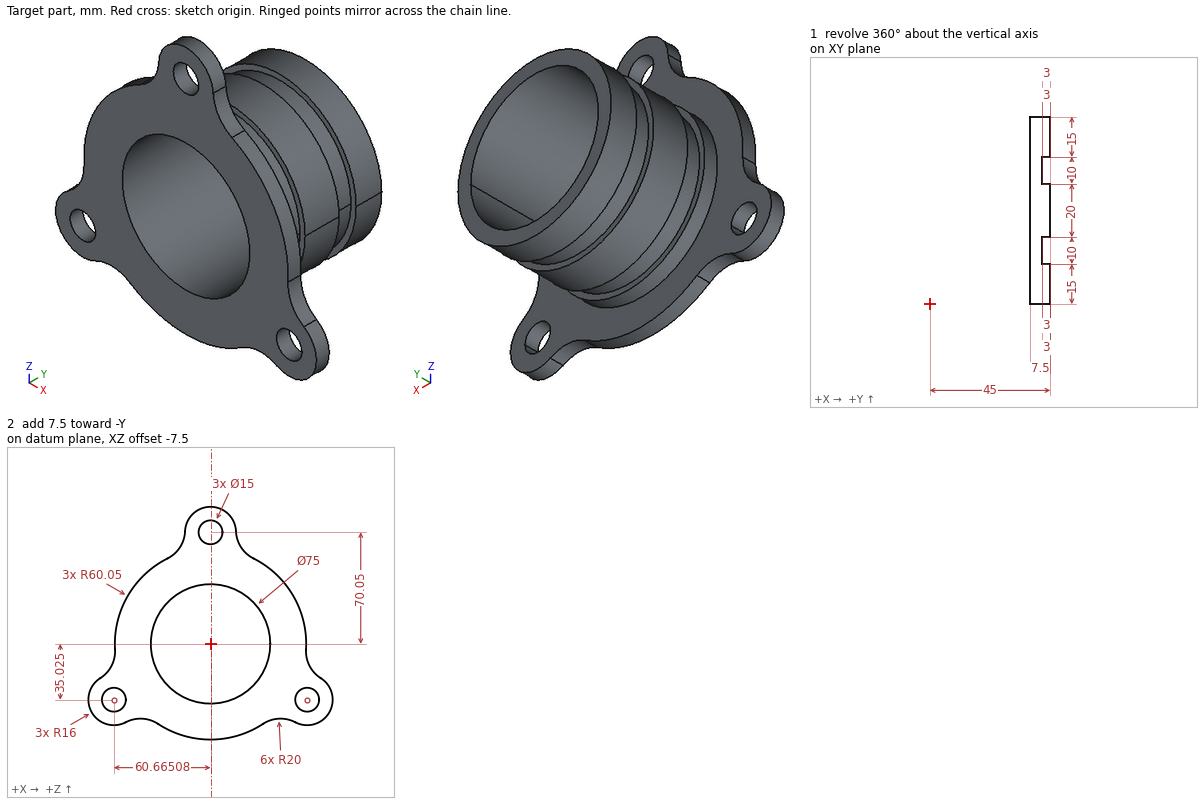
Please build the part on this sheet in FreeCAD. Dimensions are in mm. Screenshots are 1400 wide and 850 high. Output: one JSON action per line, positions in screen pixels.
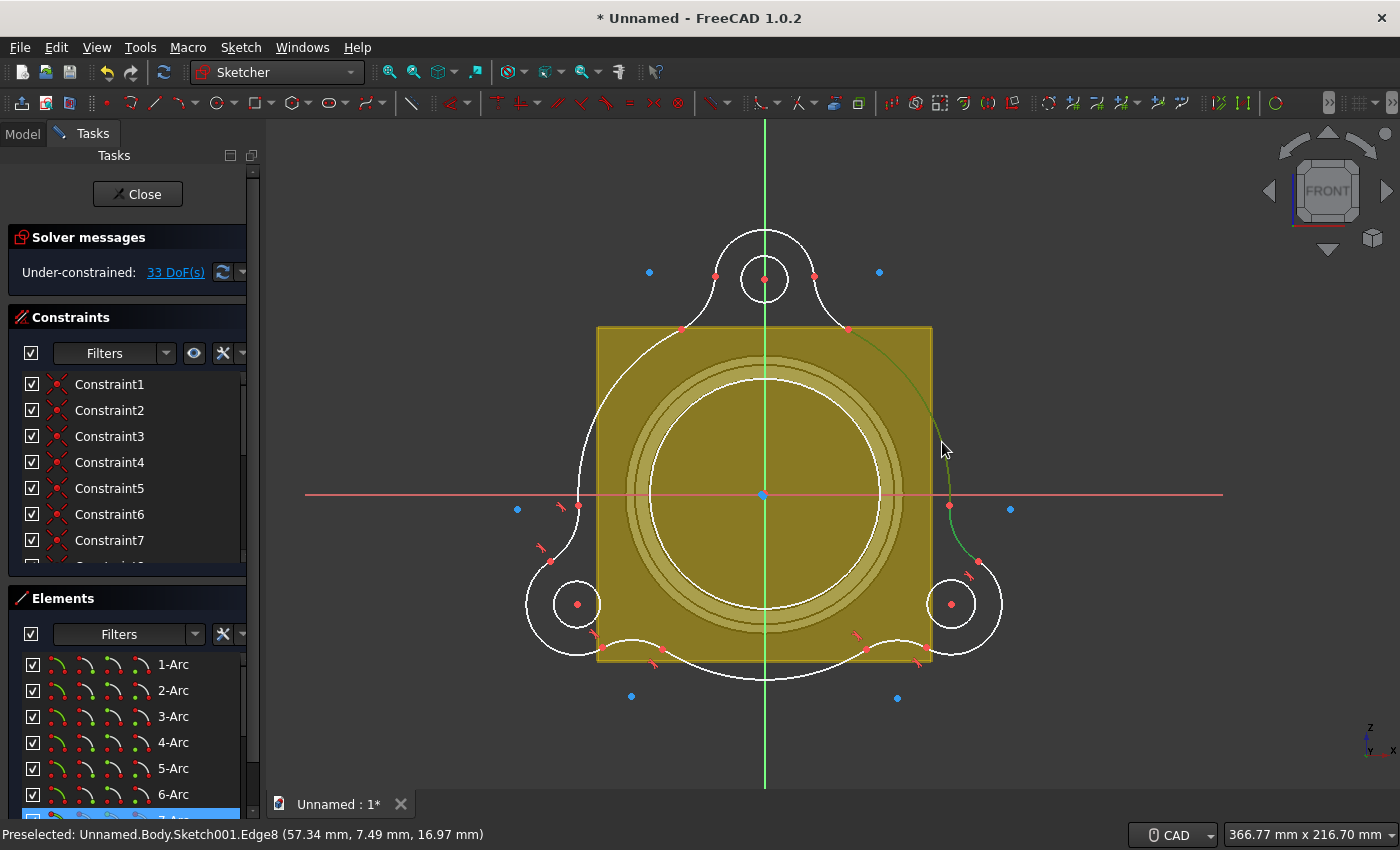
{"action": "left_click", "coordinate": [606, 104]}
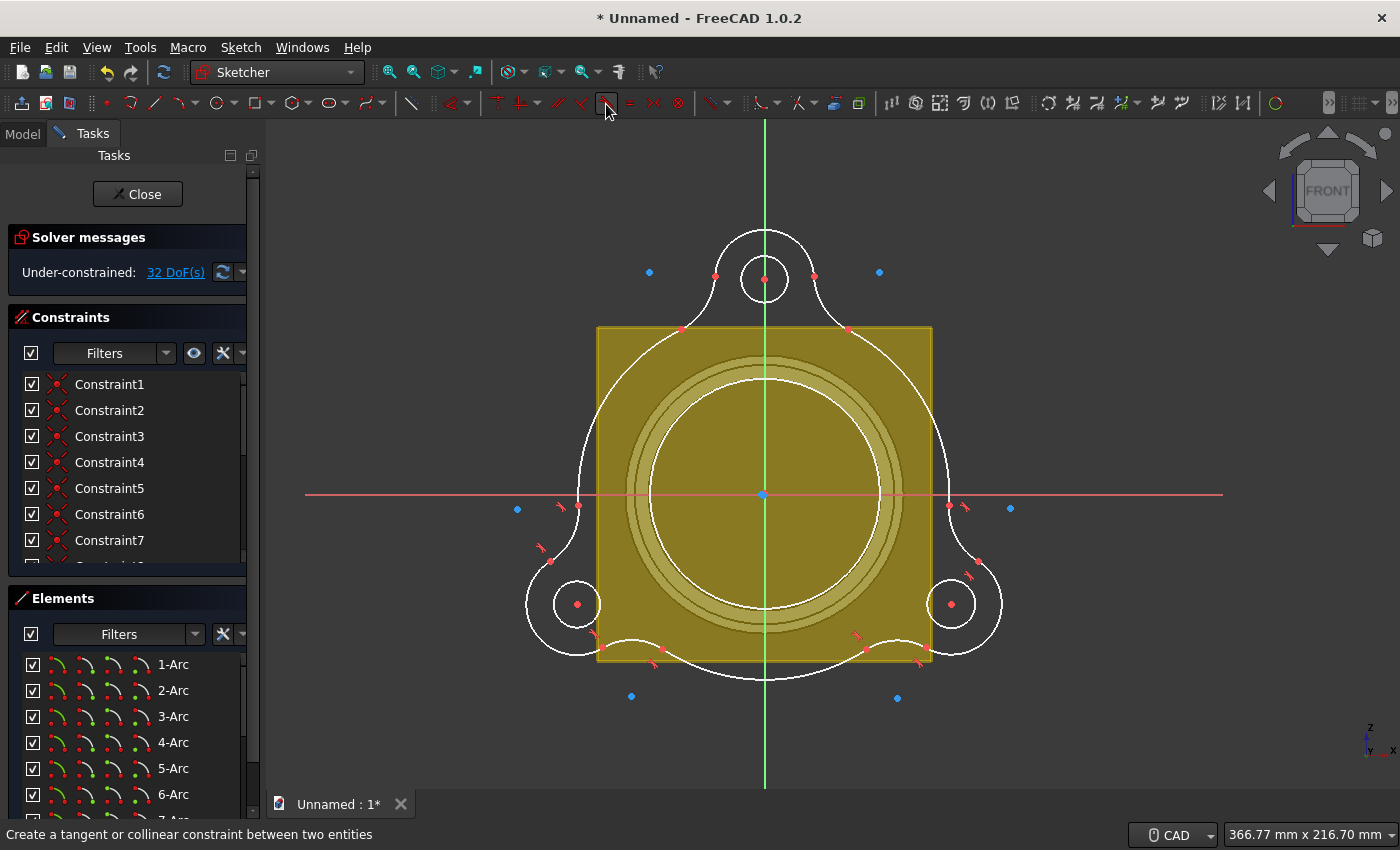
{"action": "left_click", "coordinate": [942, 442]}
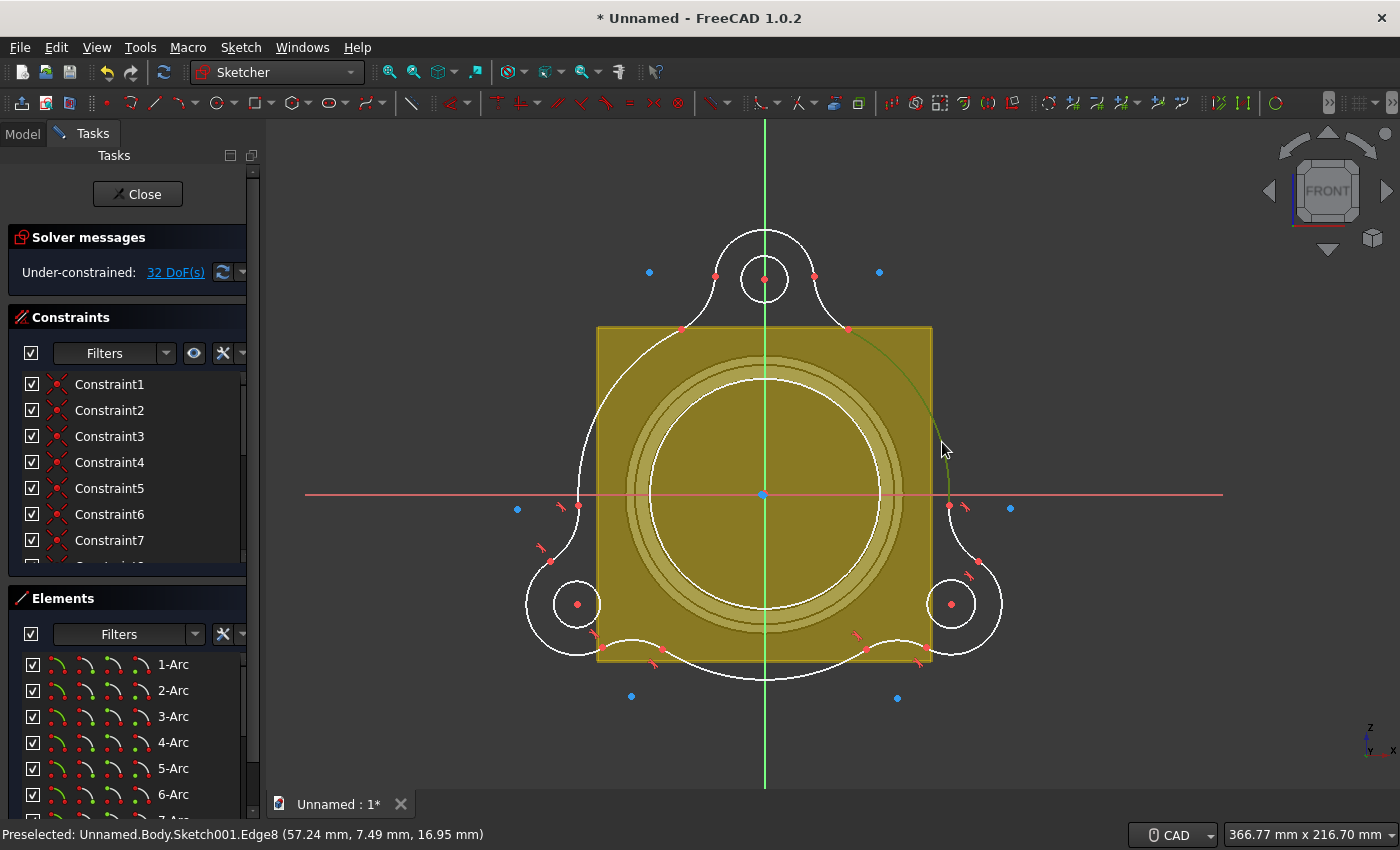
{"action": "left_click", "coordinate": [818, 296]}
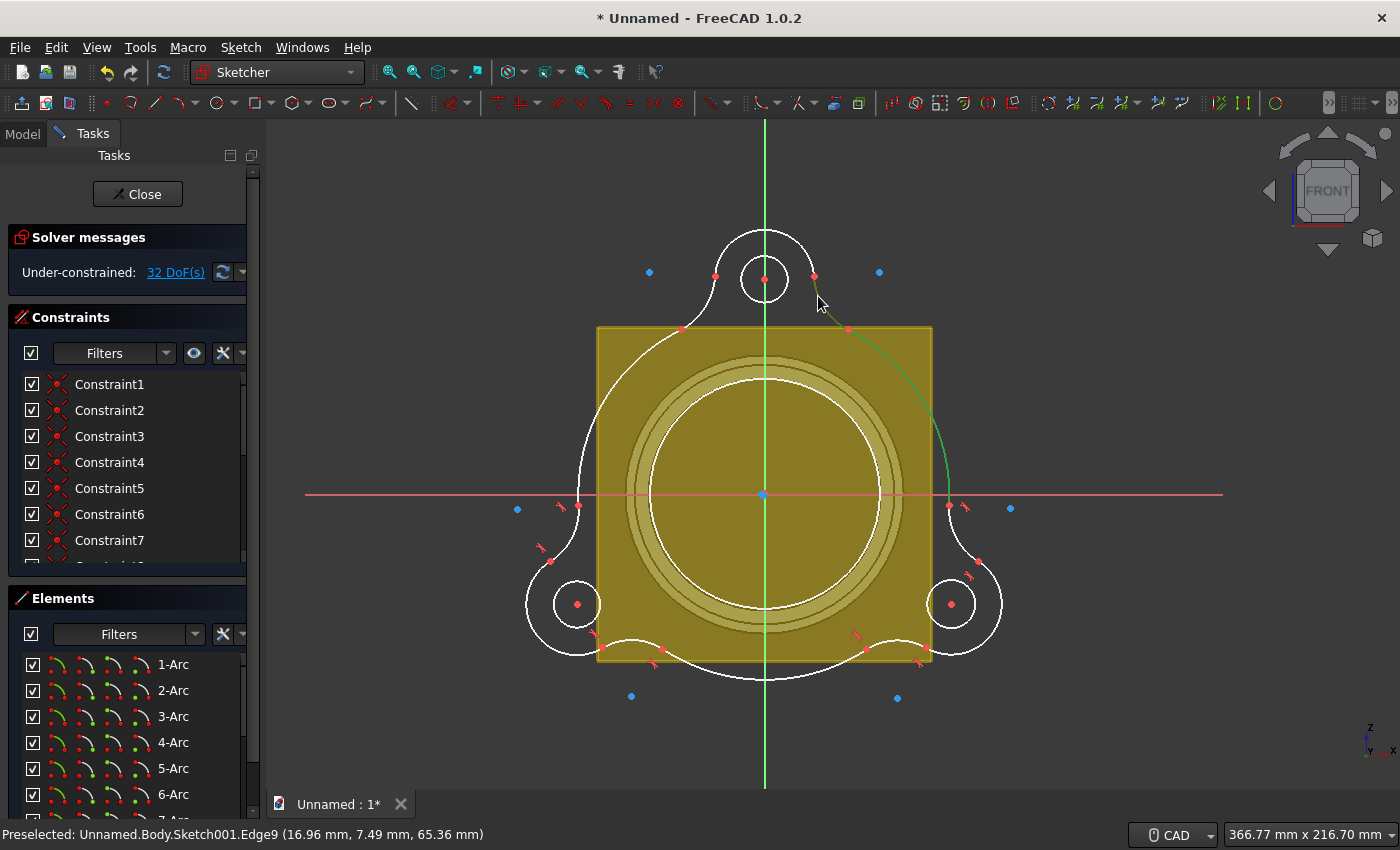
{"action": "left_click", "coordinate": [606, 104]}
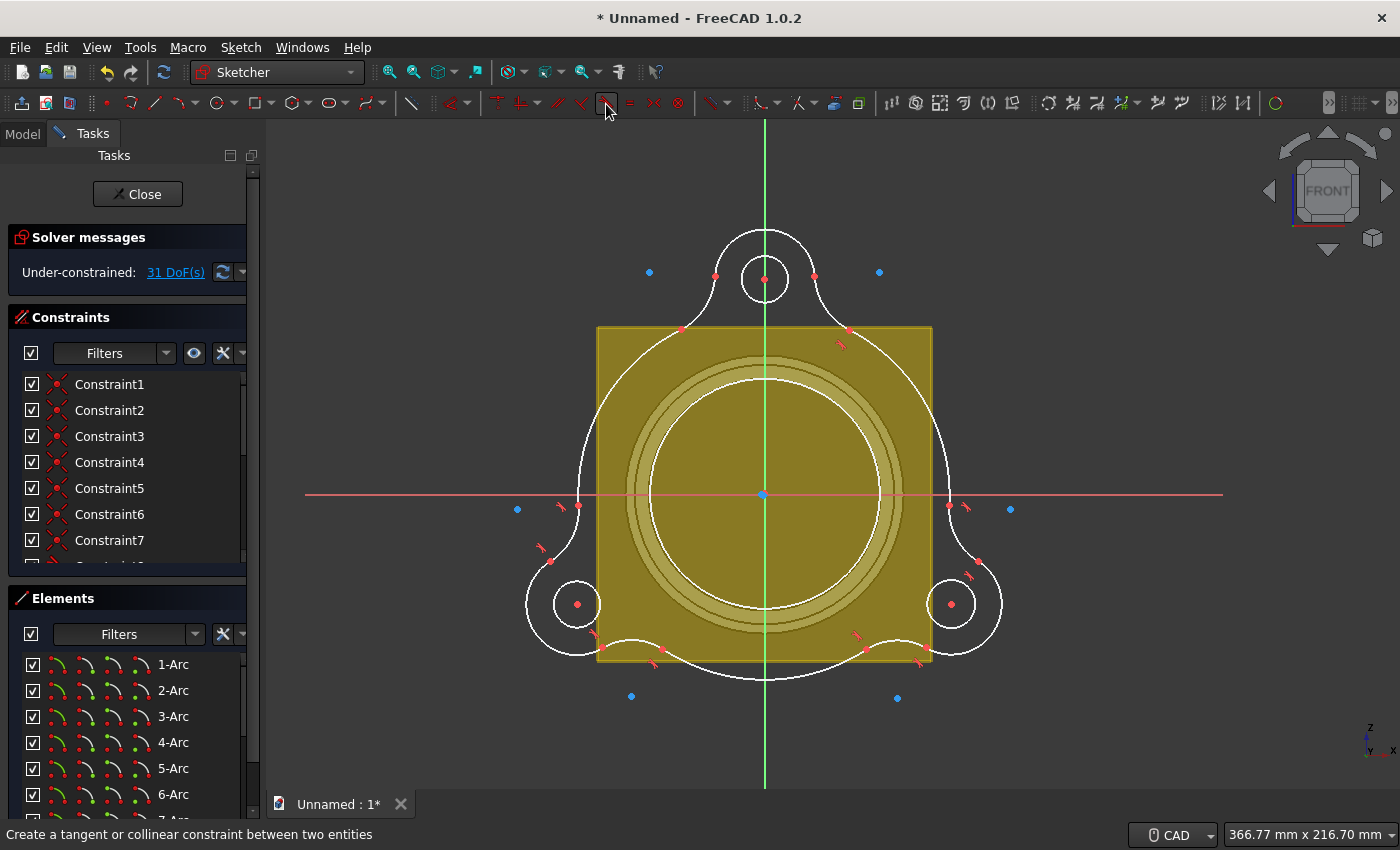
{"action": "left_click", "coordinate": [819, 296]}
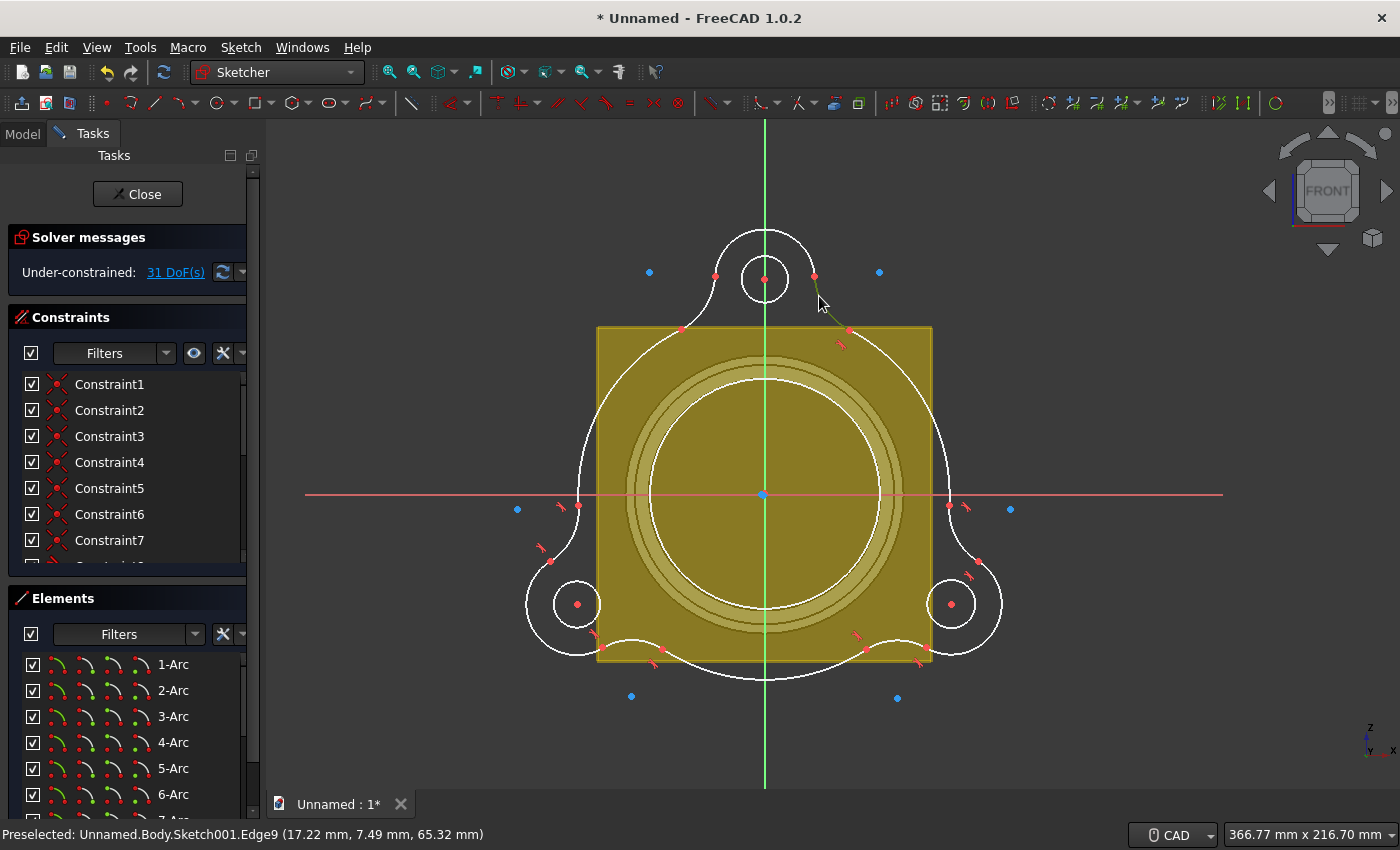
{"action": "left_click", "coordinate": [794, 239]}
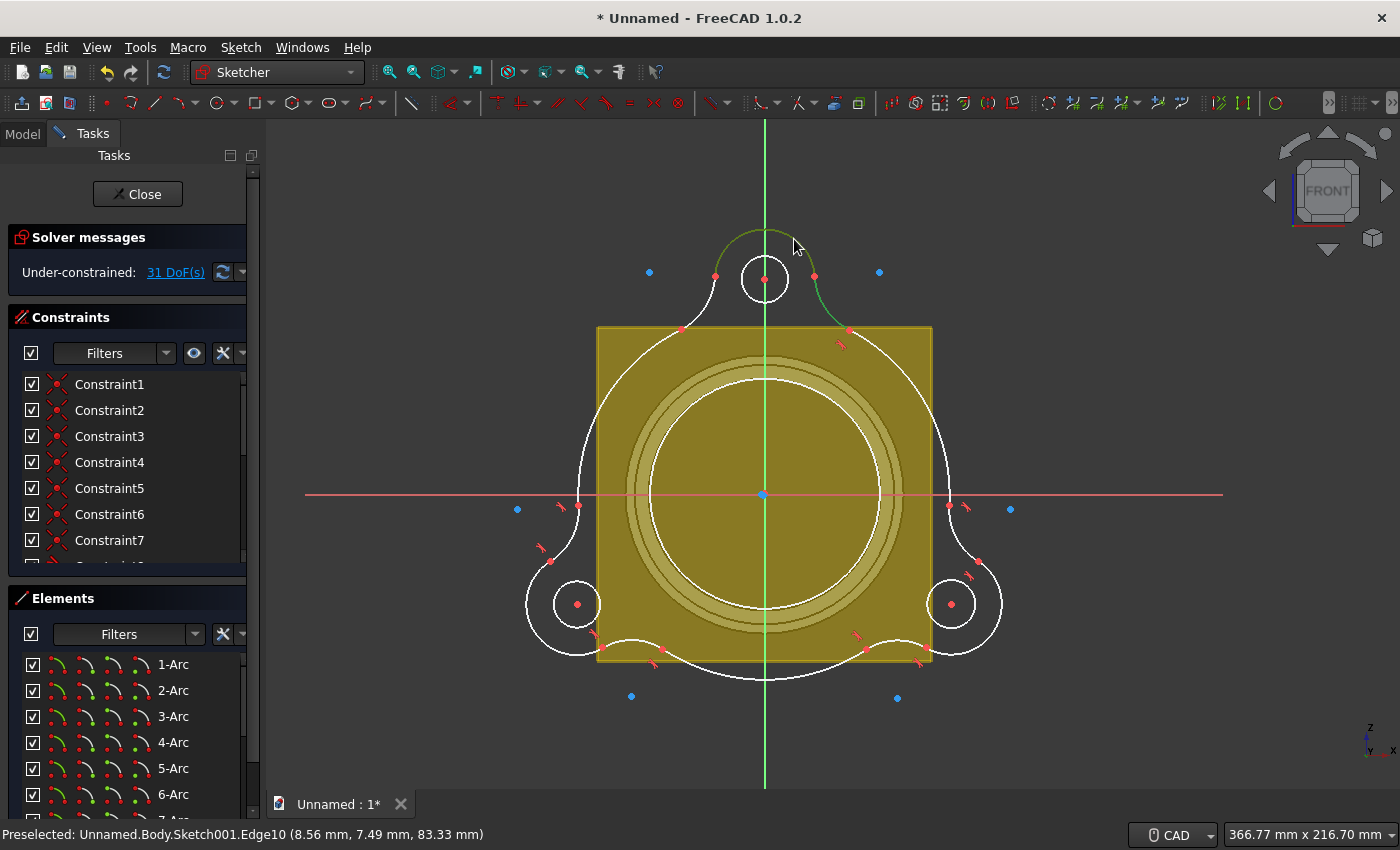
{"action": "key", "text": "t"}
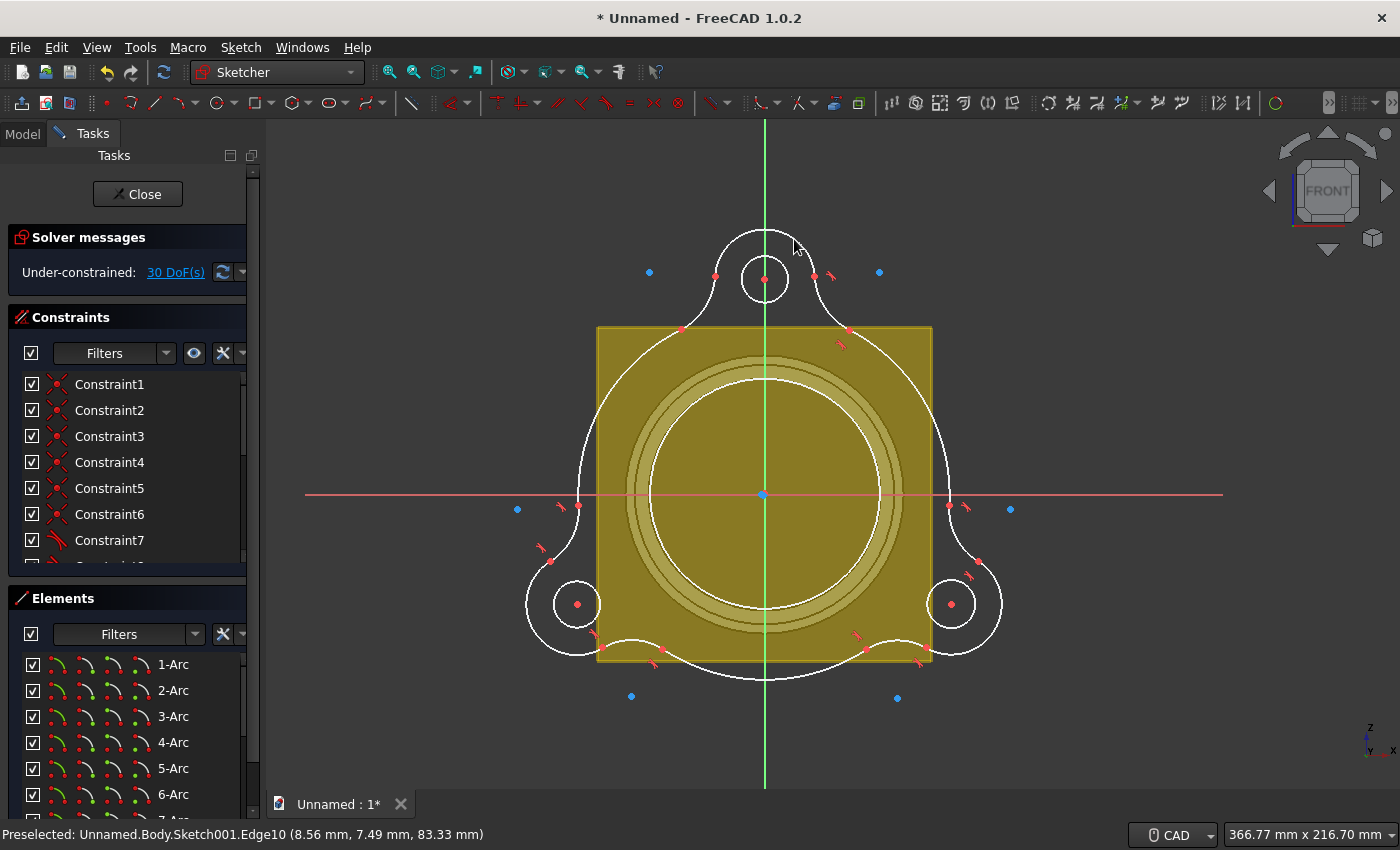
{"action": "left_click", "coordinate": [793, 238]}